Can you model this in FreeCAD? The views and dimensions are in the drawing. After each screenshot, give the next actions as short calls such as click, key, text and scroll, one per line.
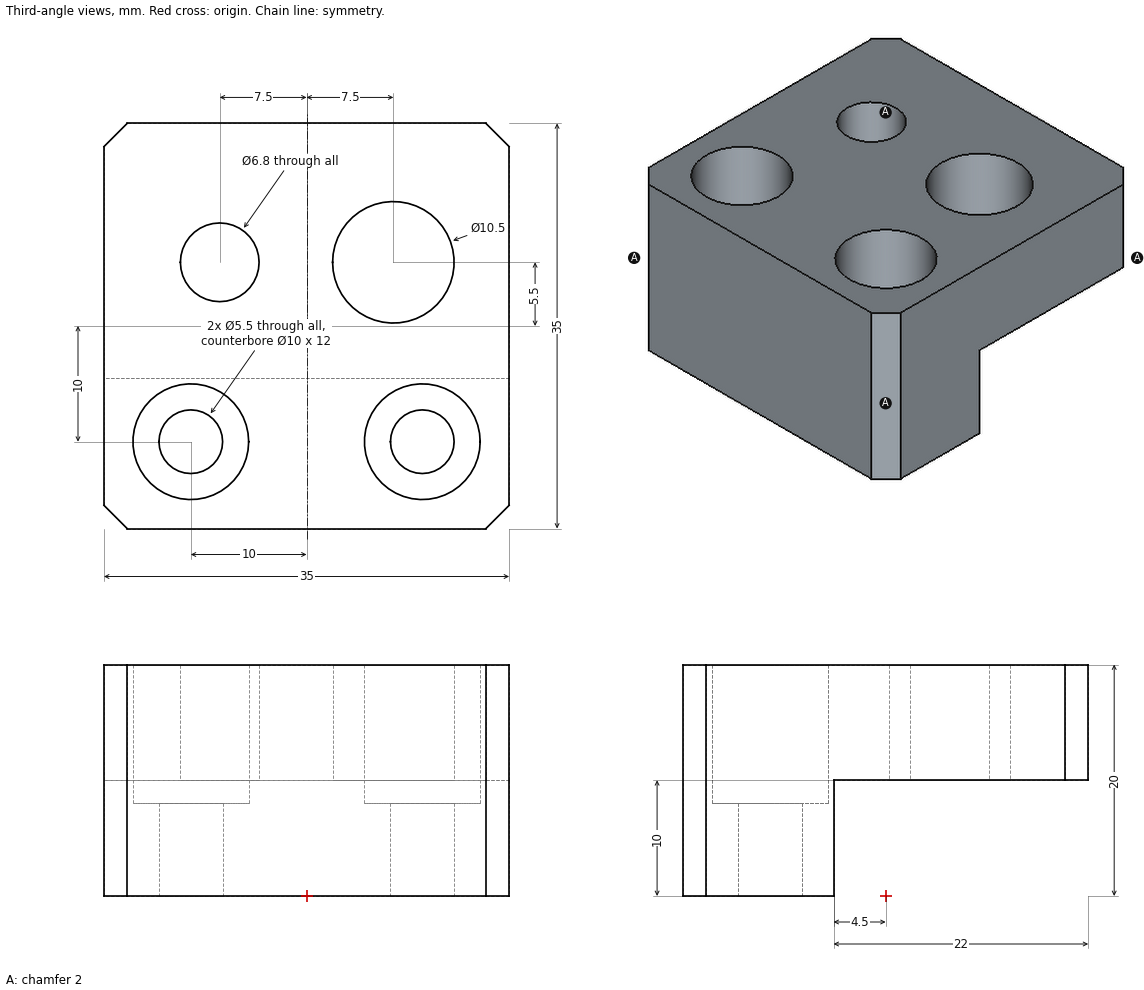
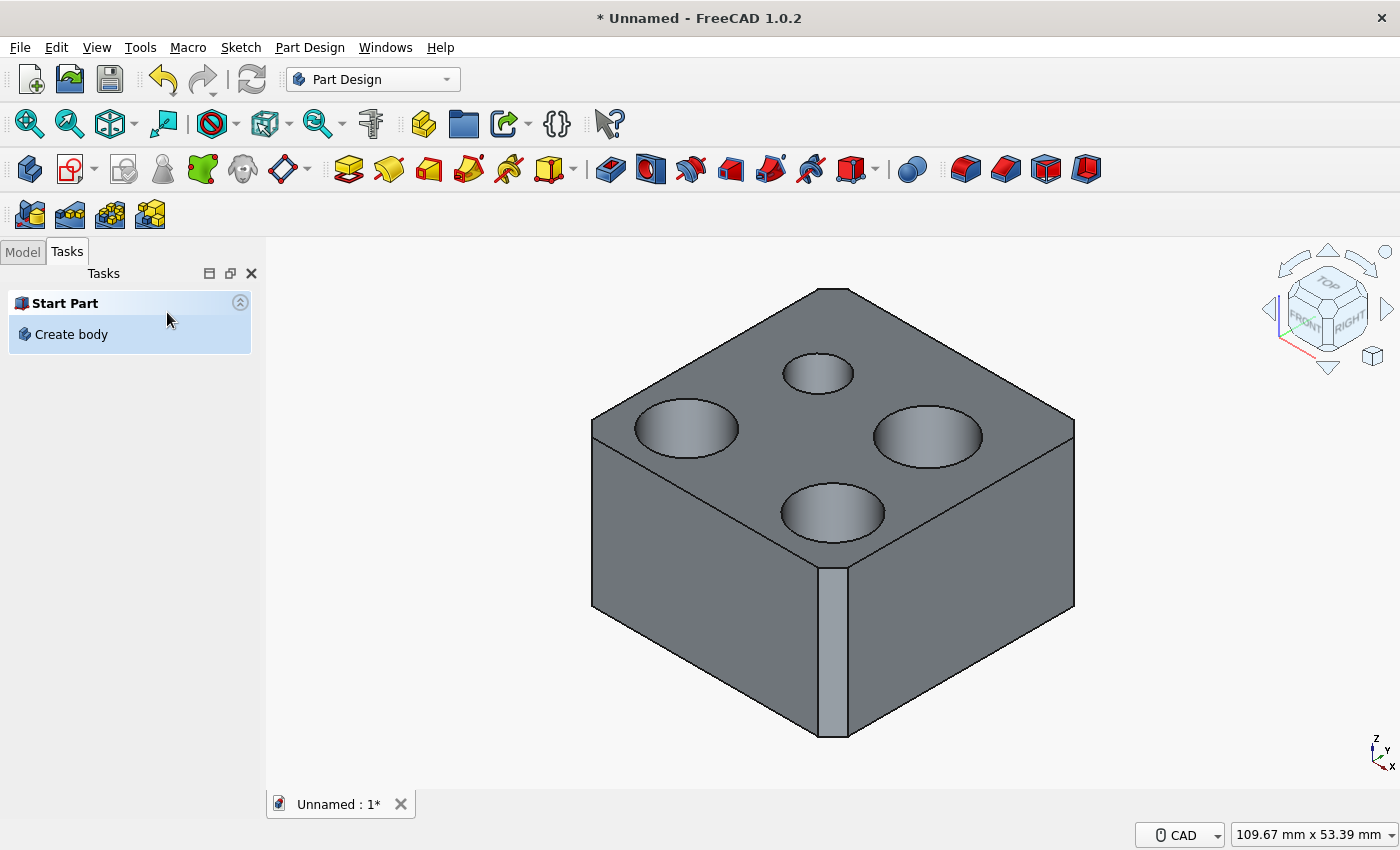
click(993, 567)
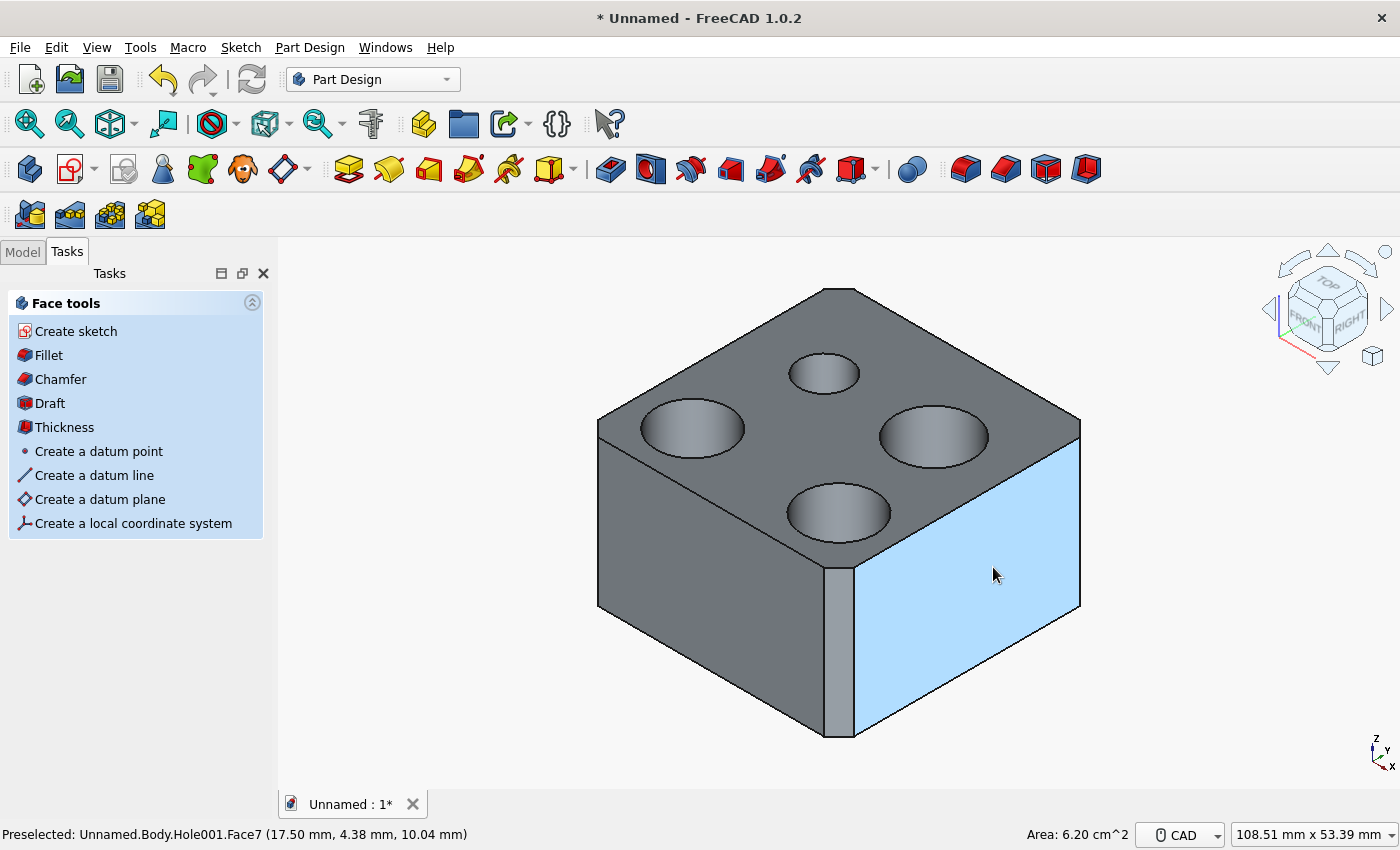
click(70, 170)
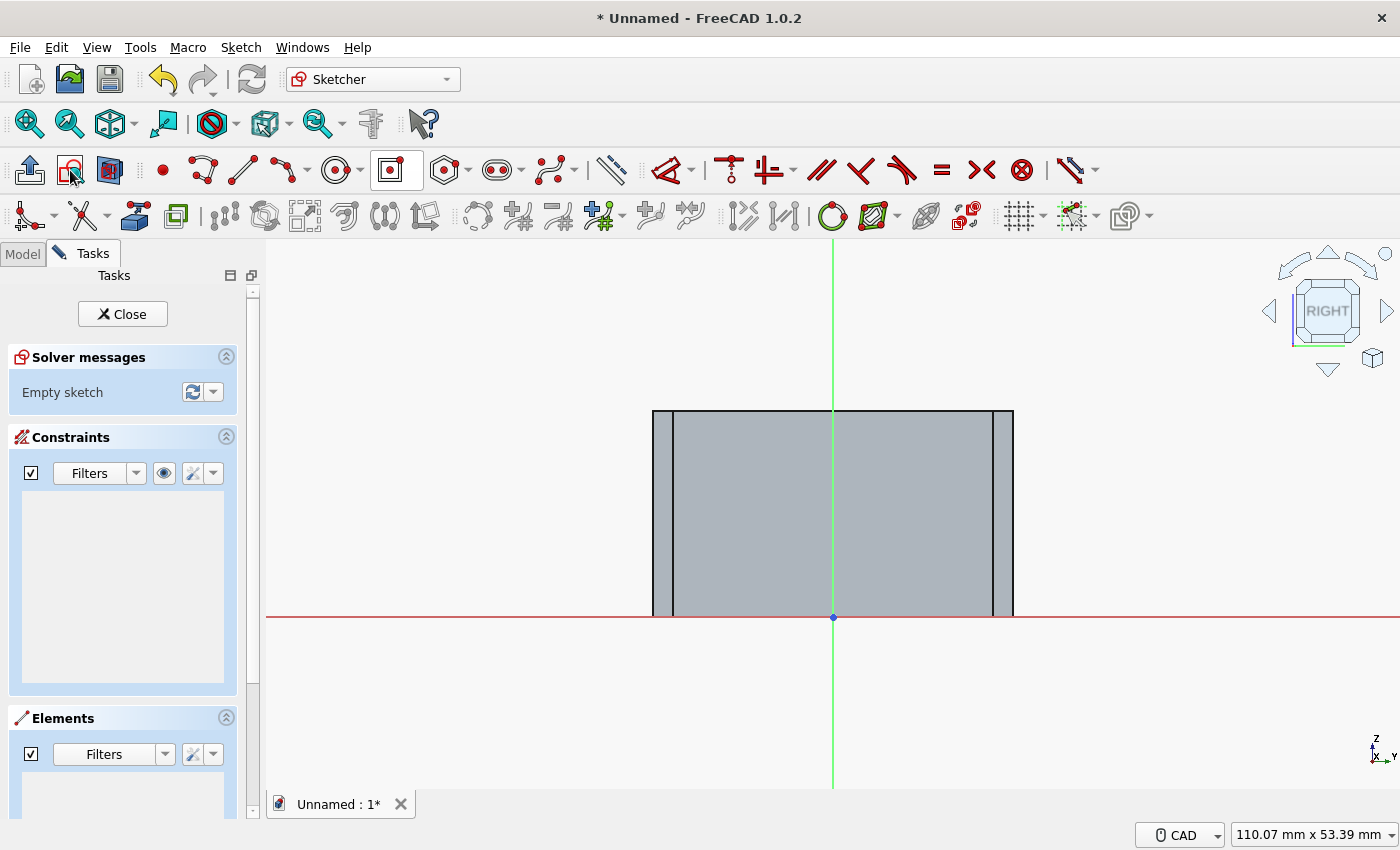
scroll(979, 595, up, 5)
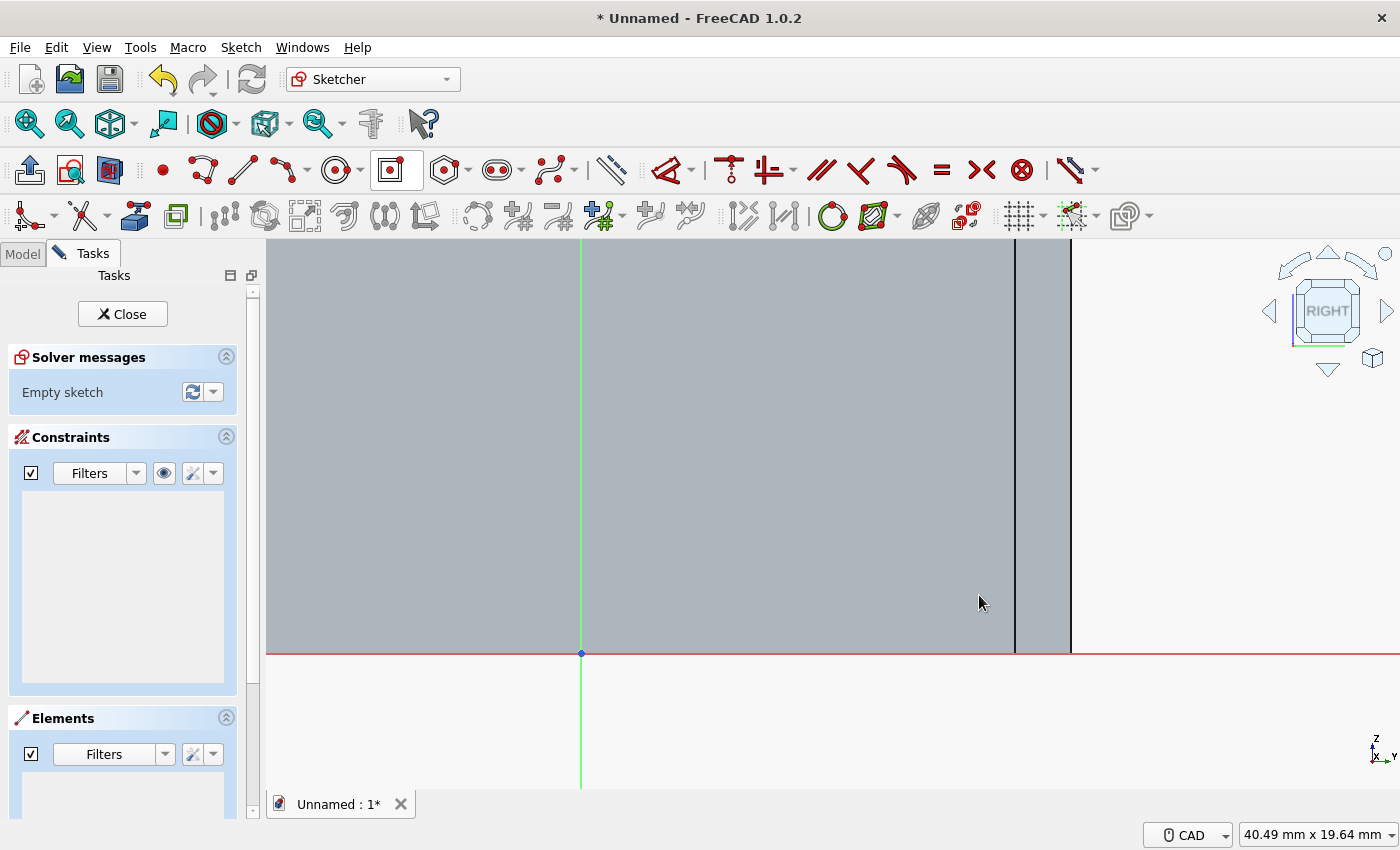
click(418, 170)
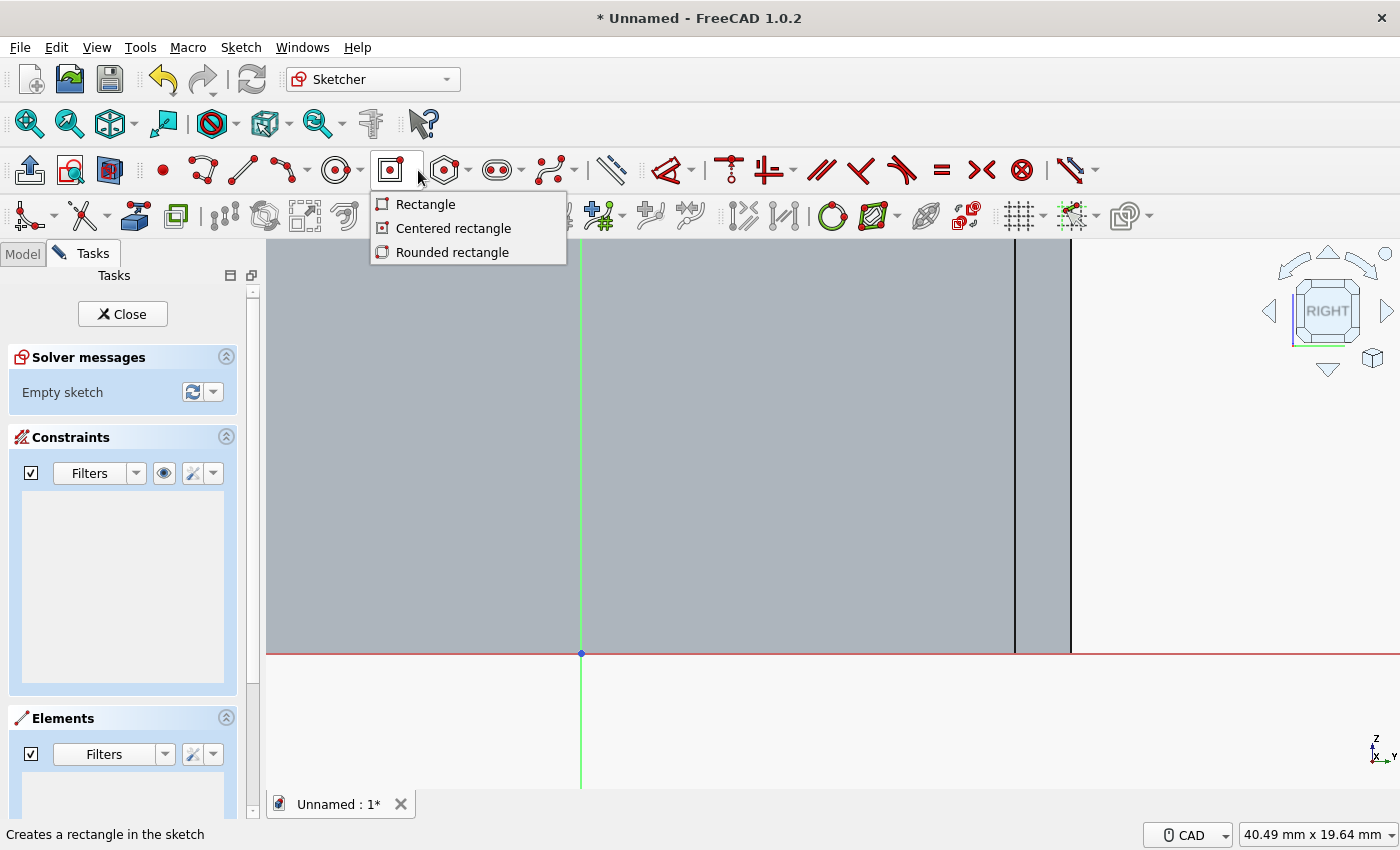
click(468, 204)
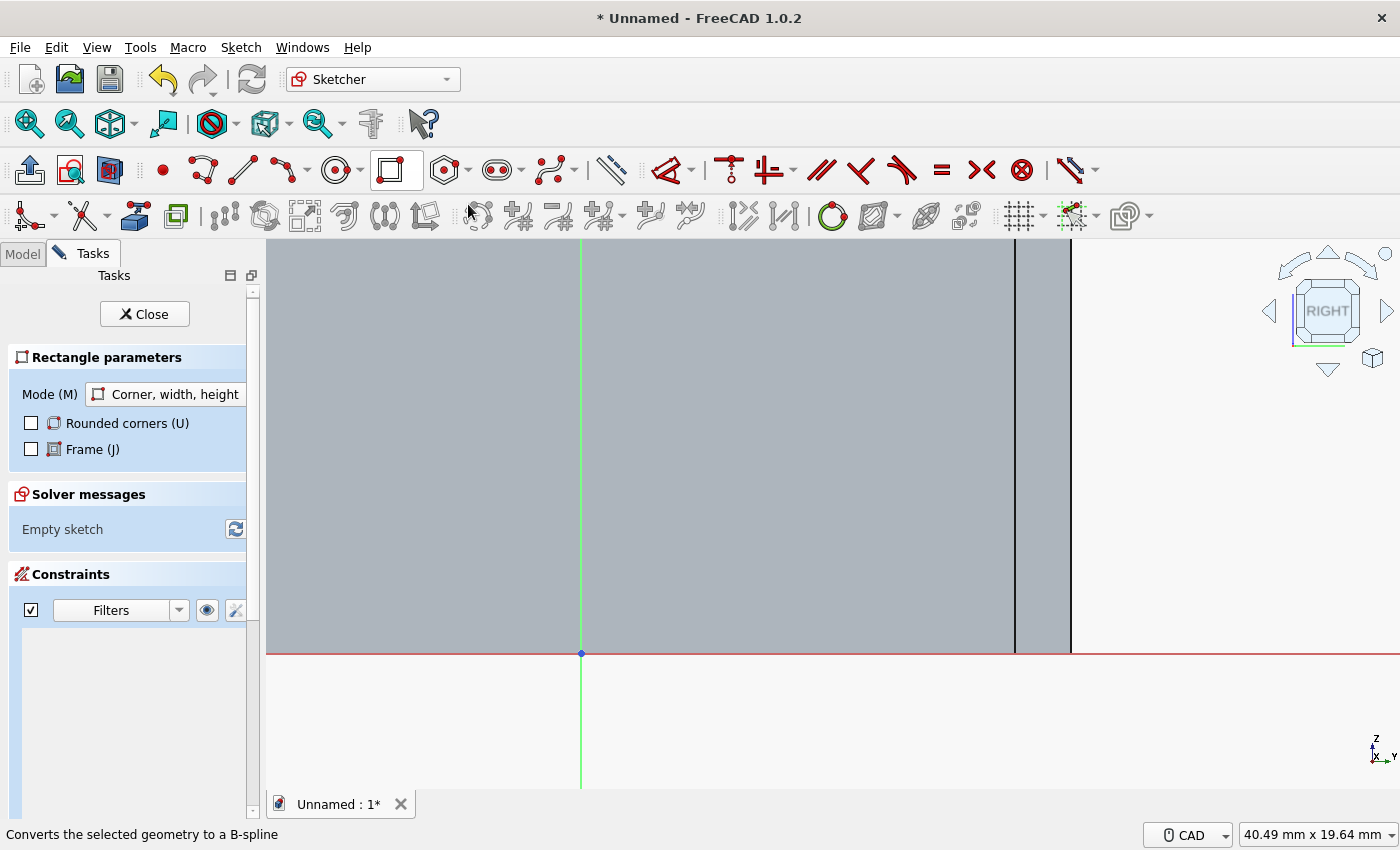
click(455, 374)
click(1071, 654)
key(Escape)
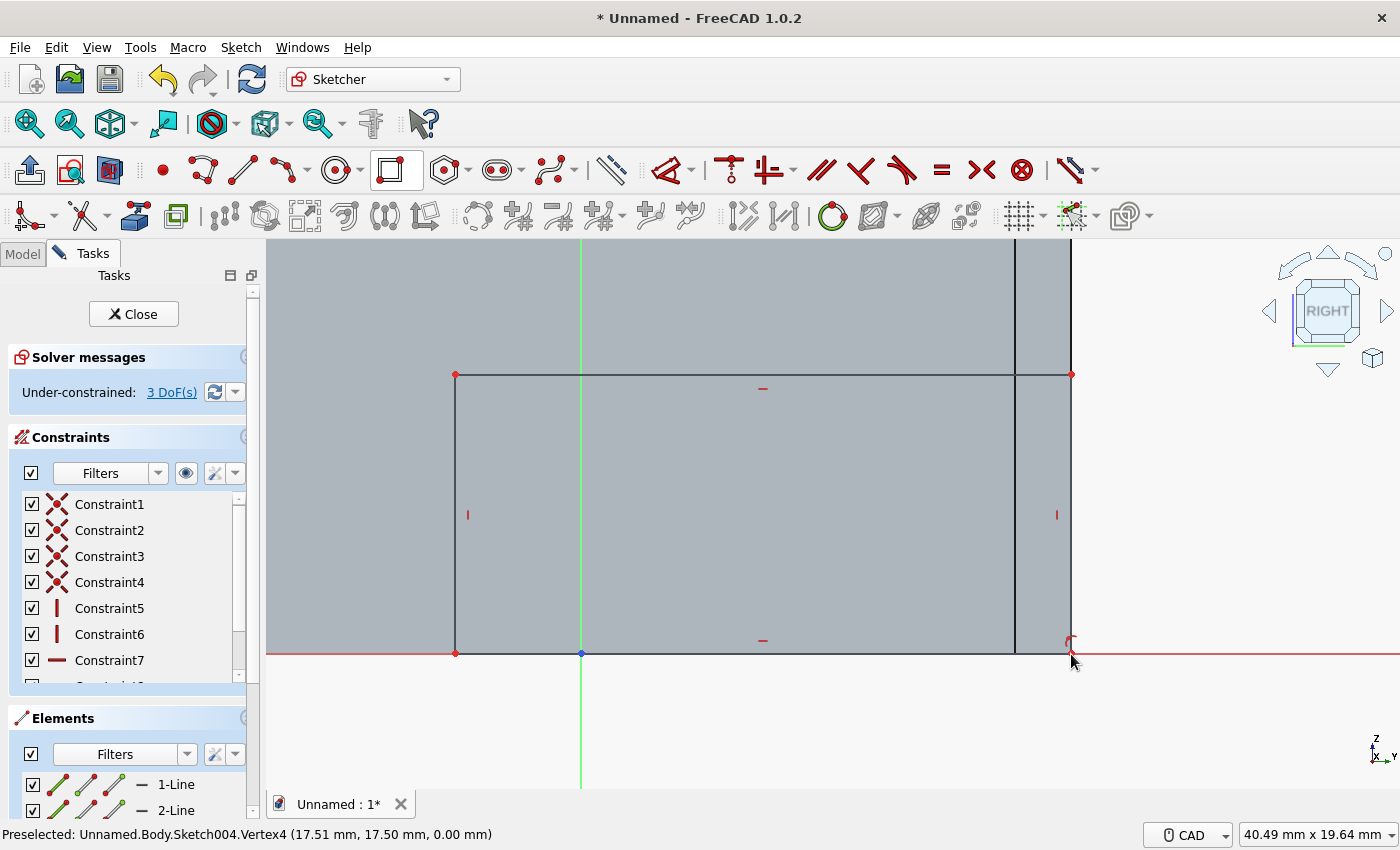
key(d)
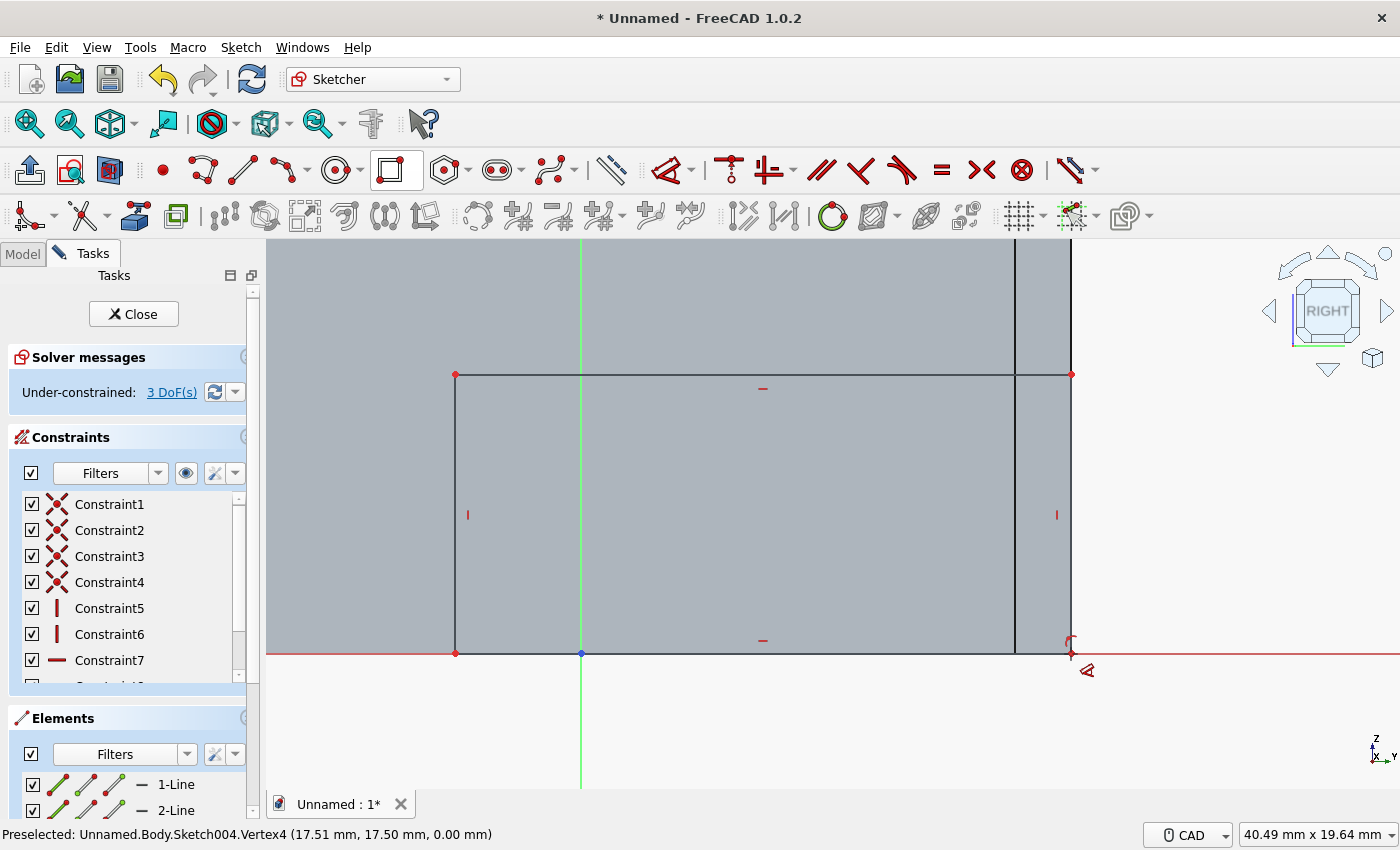
click(455, 459)
click(421, 514)